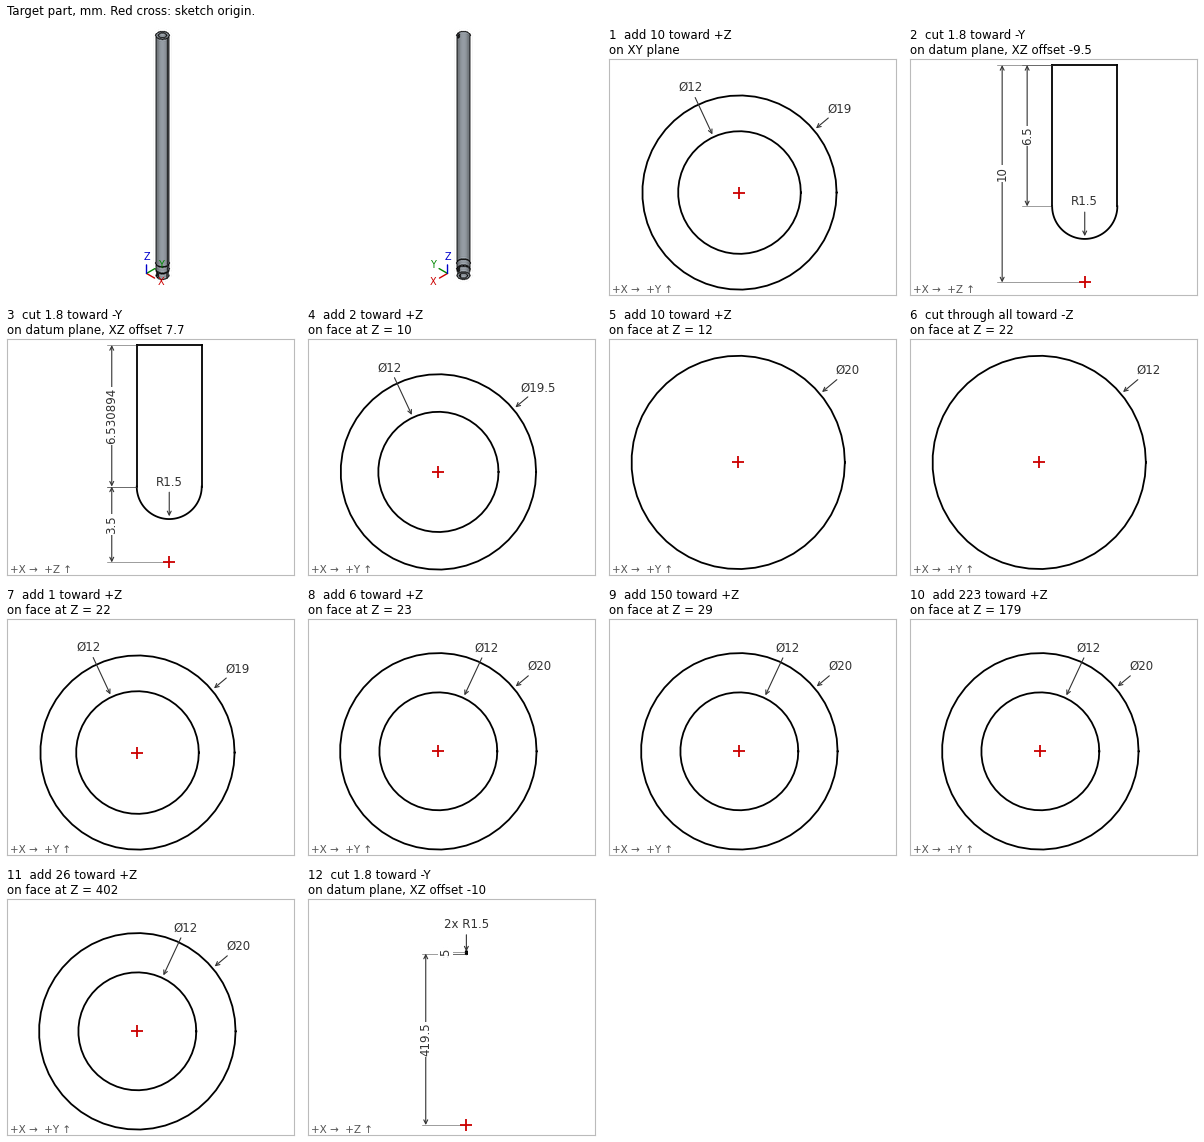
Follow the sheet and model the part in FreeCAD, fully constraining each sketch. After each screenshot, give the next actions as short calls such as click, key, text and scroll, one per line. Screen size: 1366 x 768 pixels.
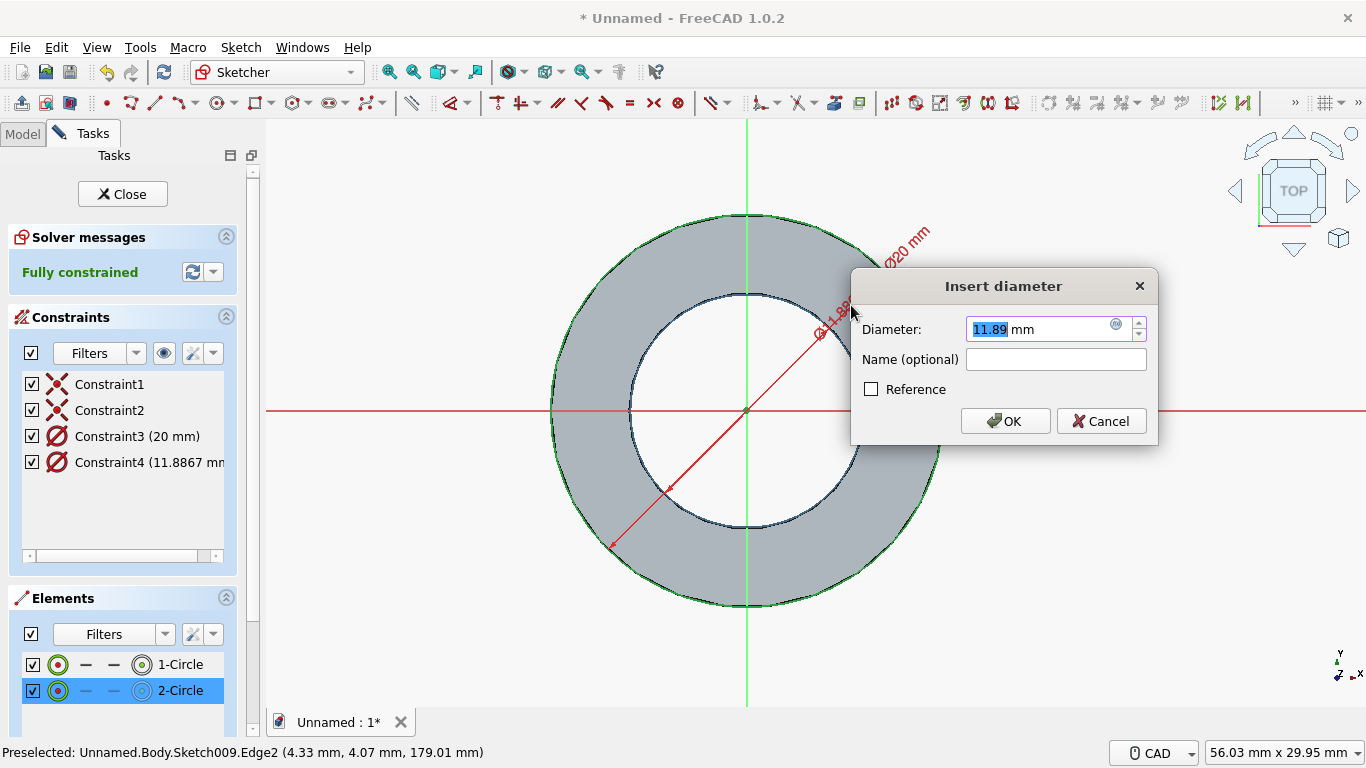
text(12)
key(Return)
key(Escape)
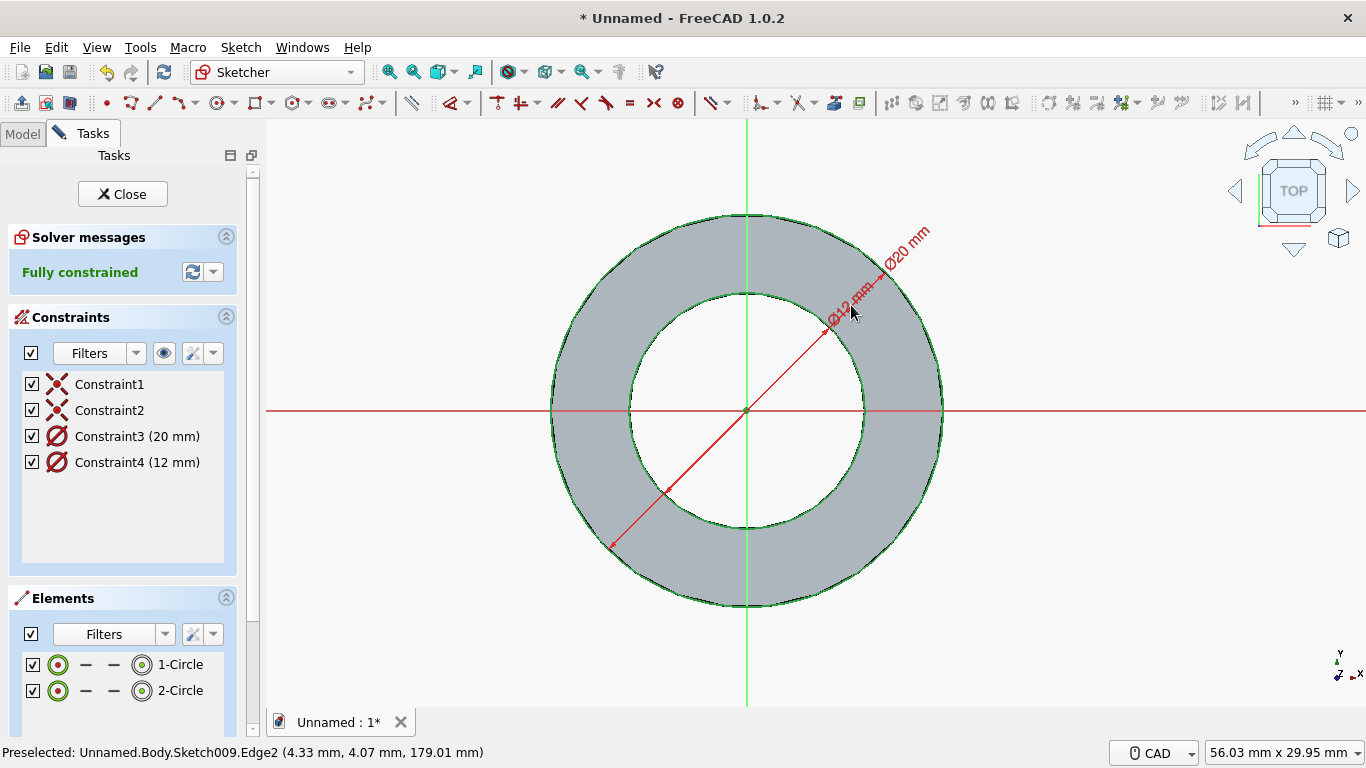
click(123, 194)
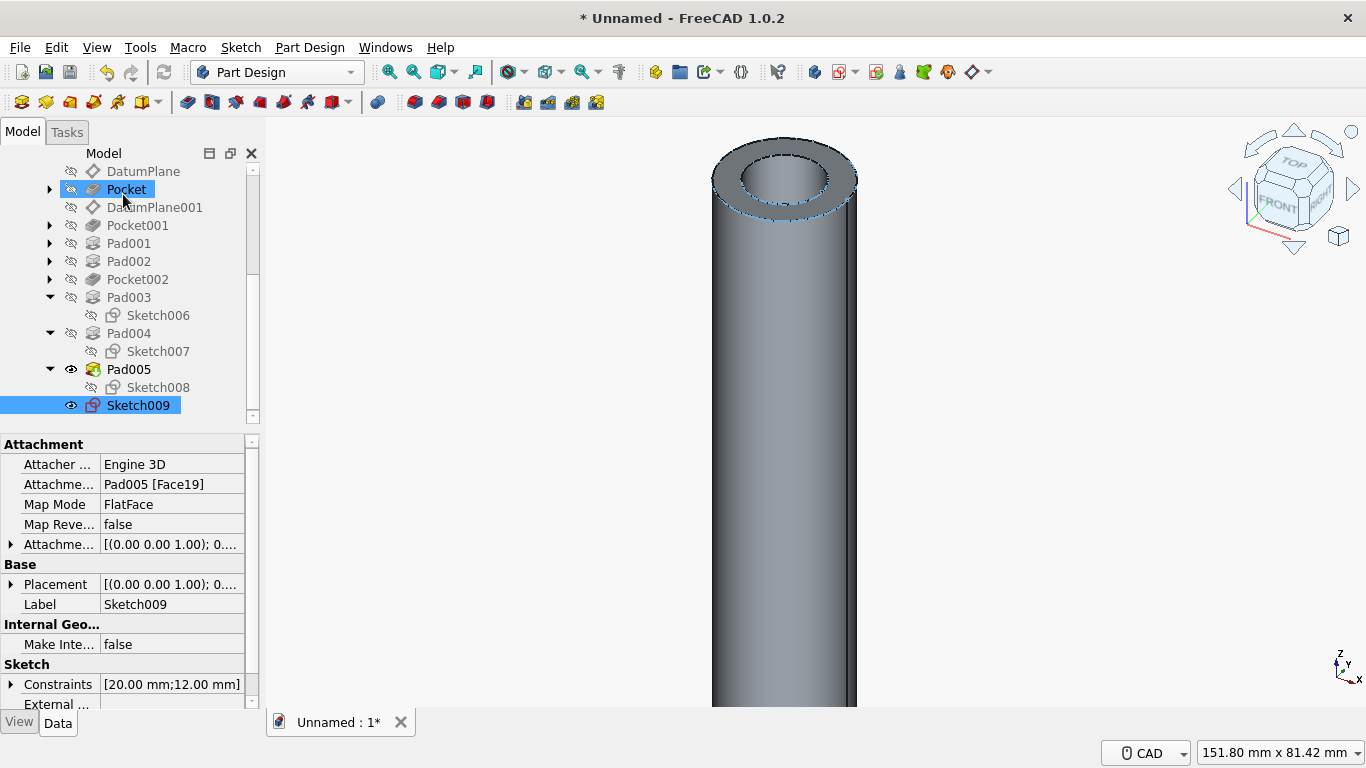
click(22, 102)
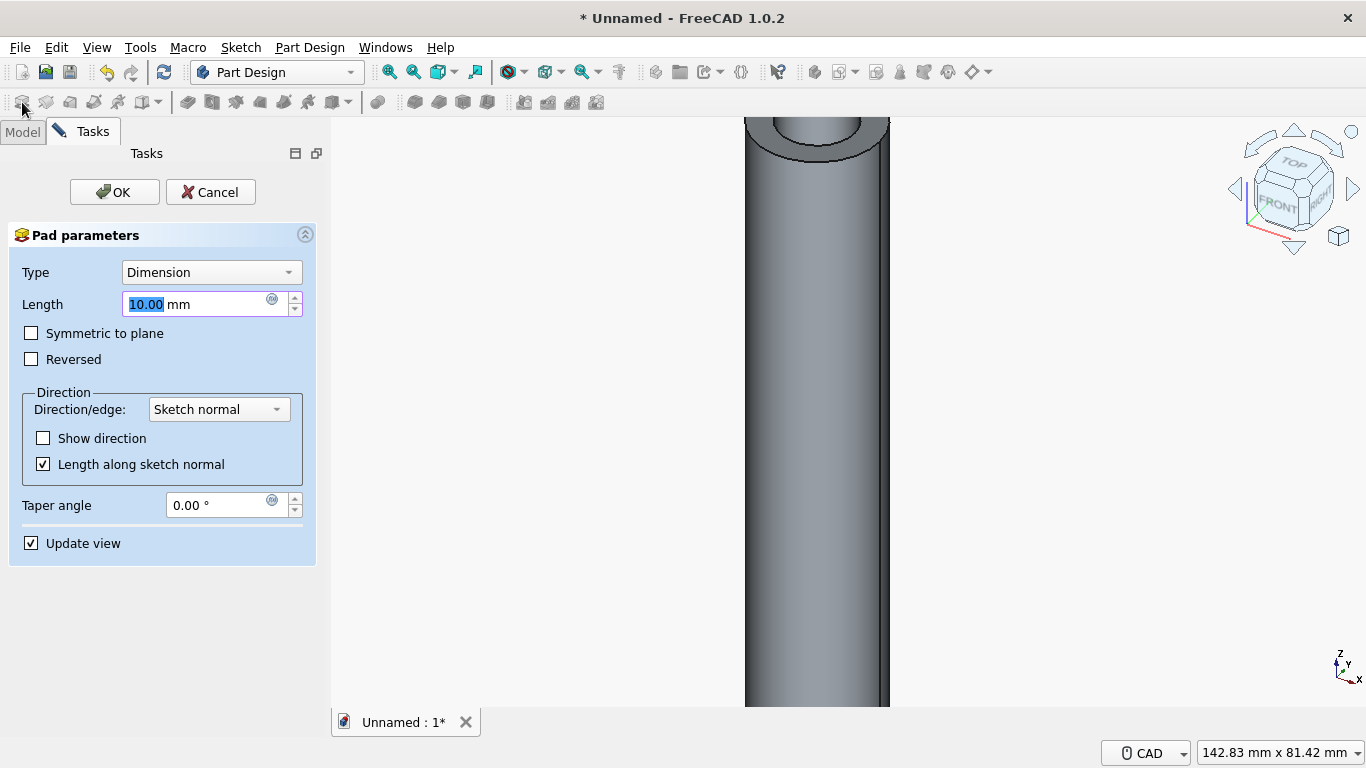
text(223)
key(Tab)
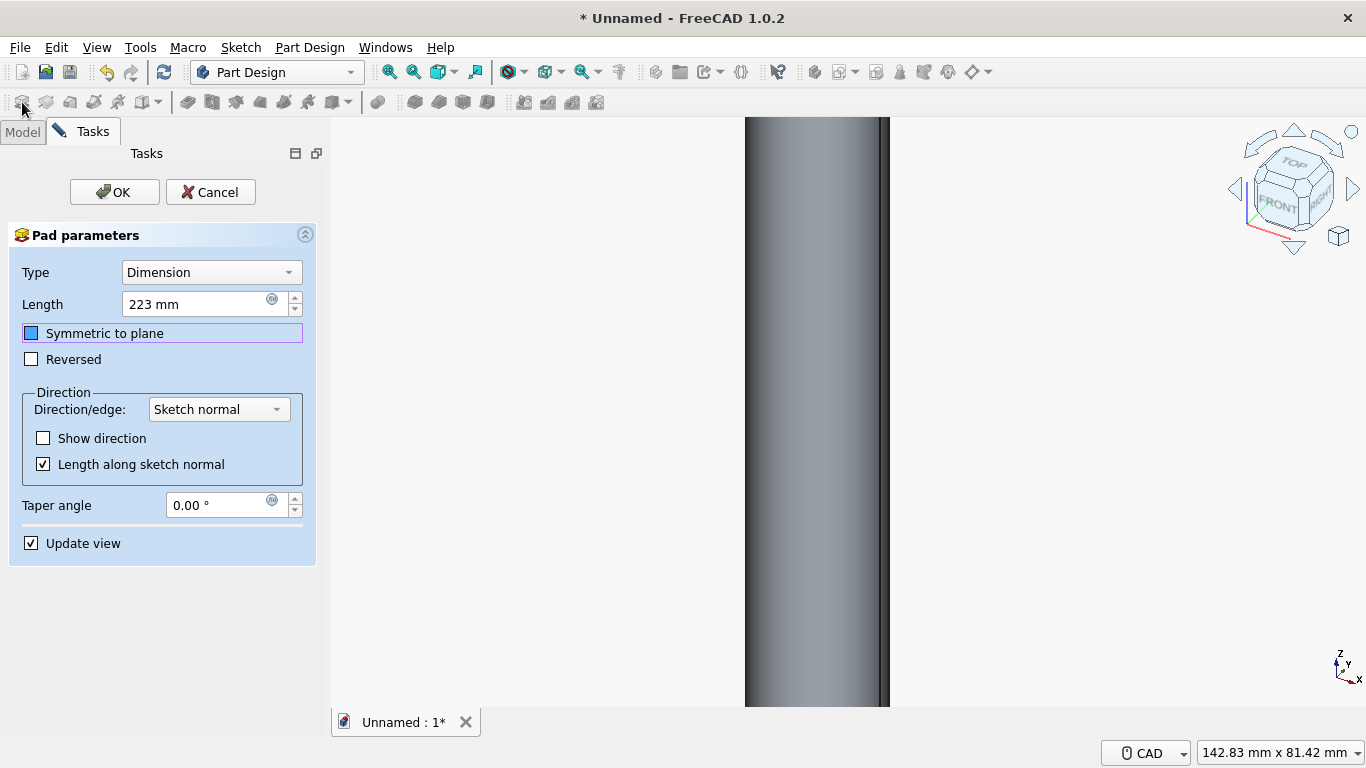
click(115, 192)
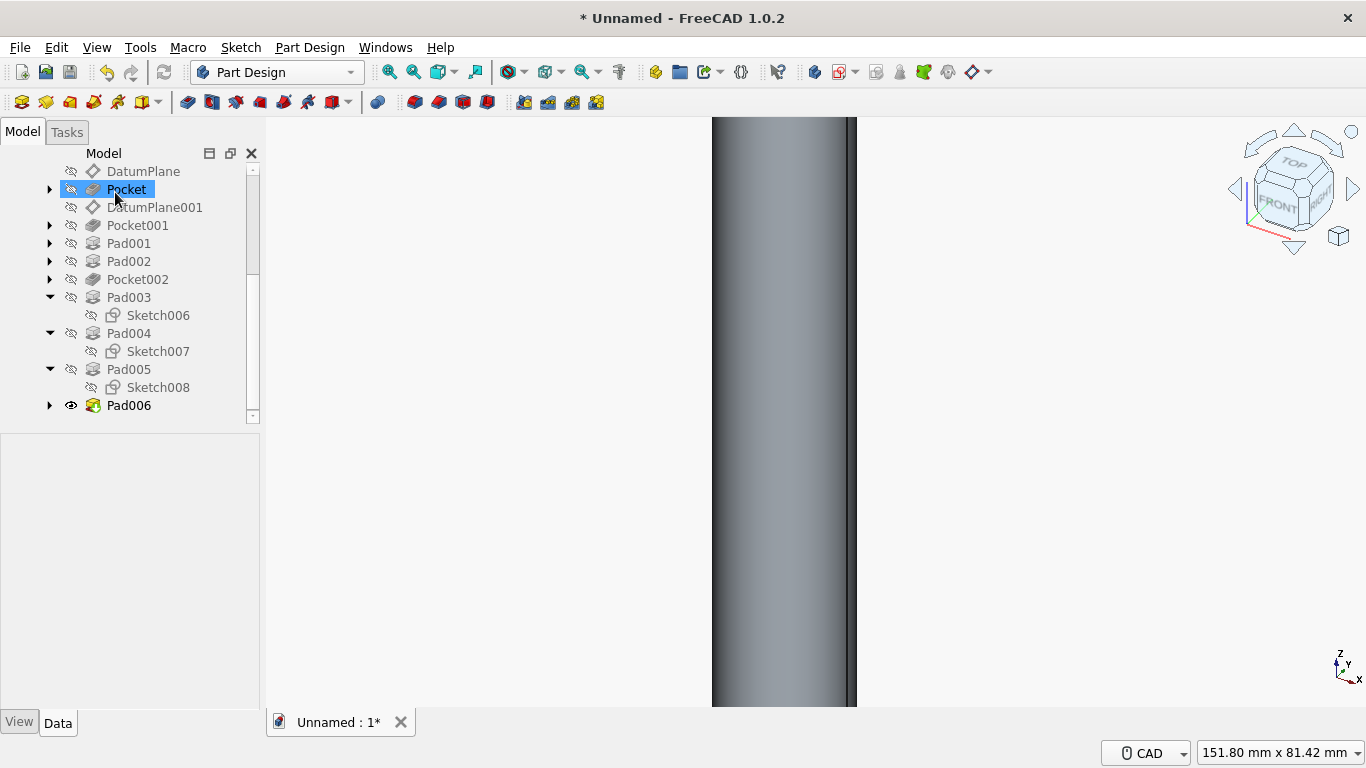
click(390, 72)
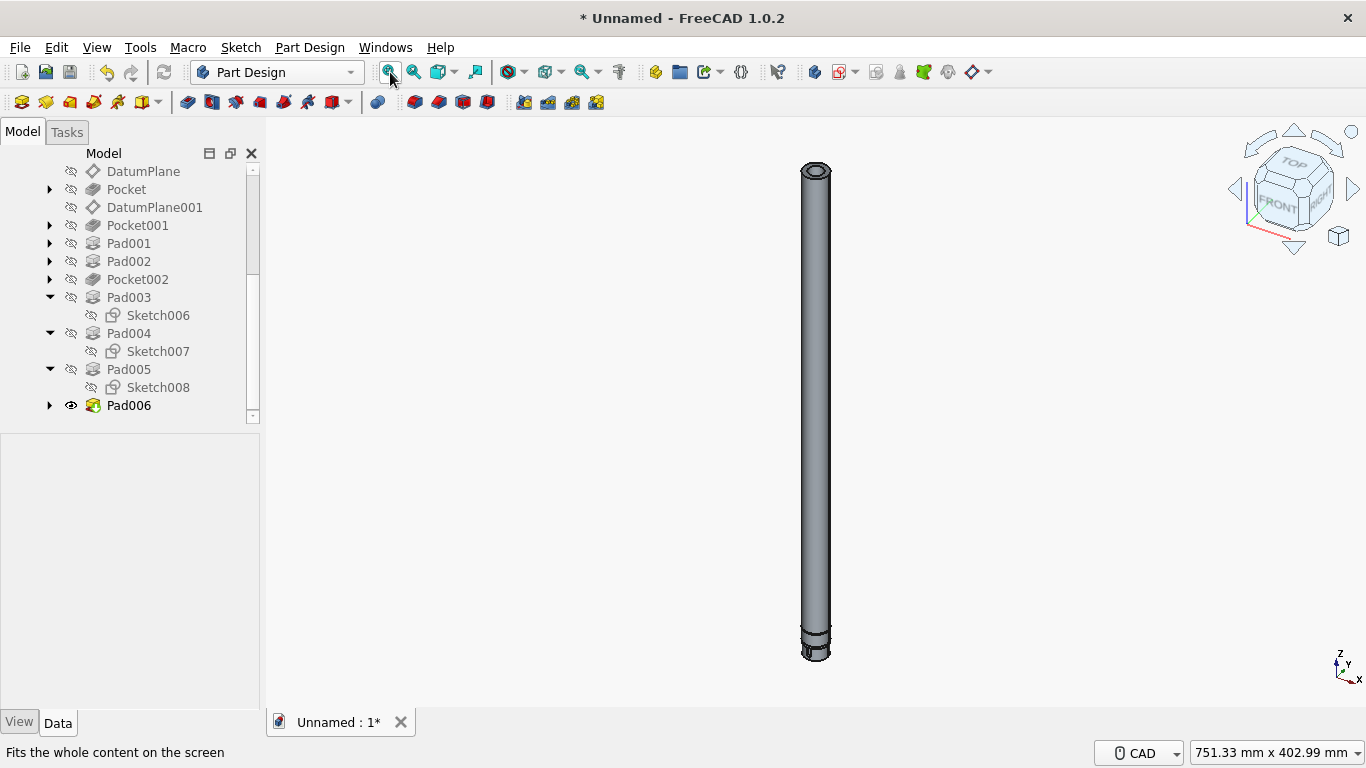
scroll(827, 168, up, 8)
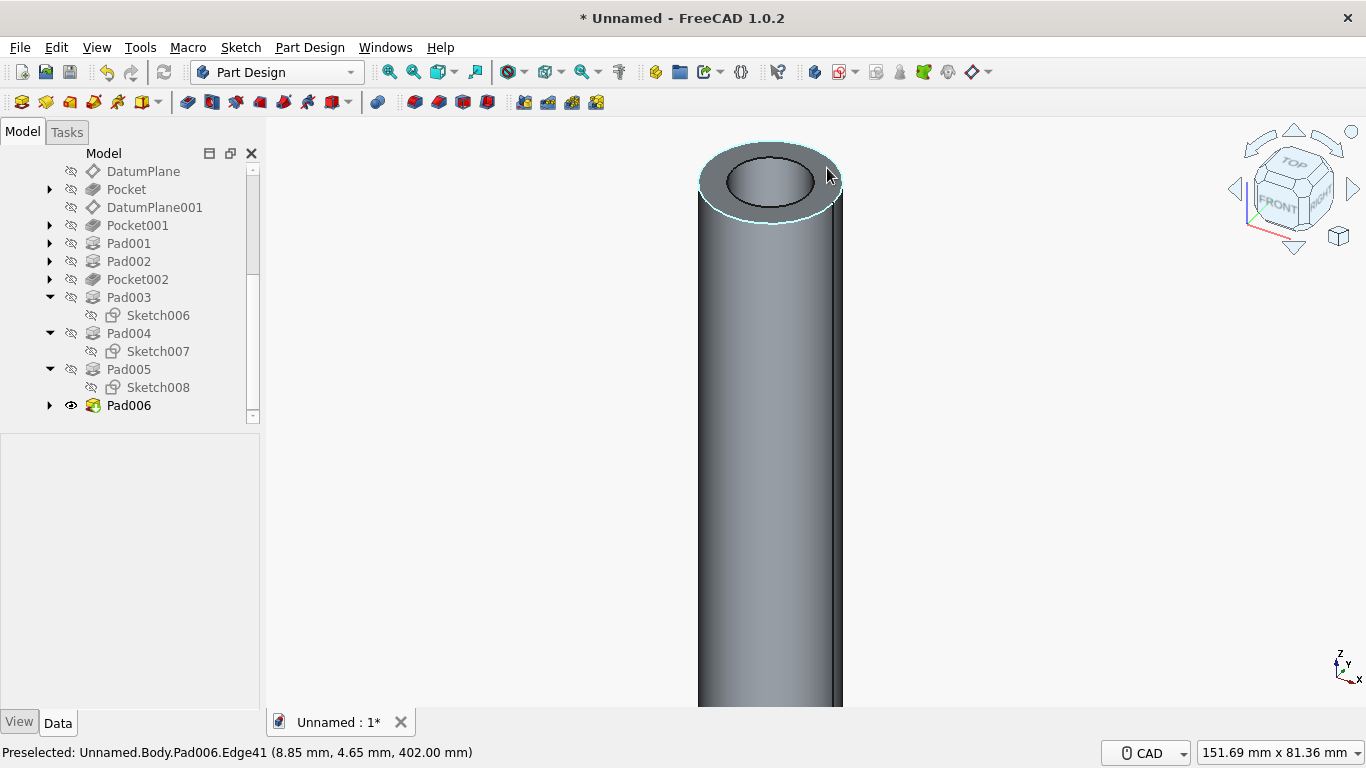
click(827, 173)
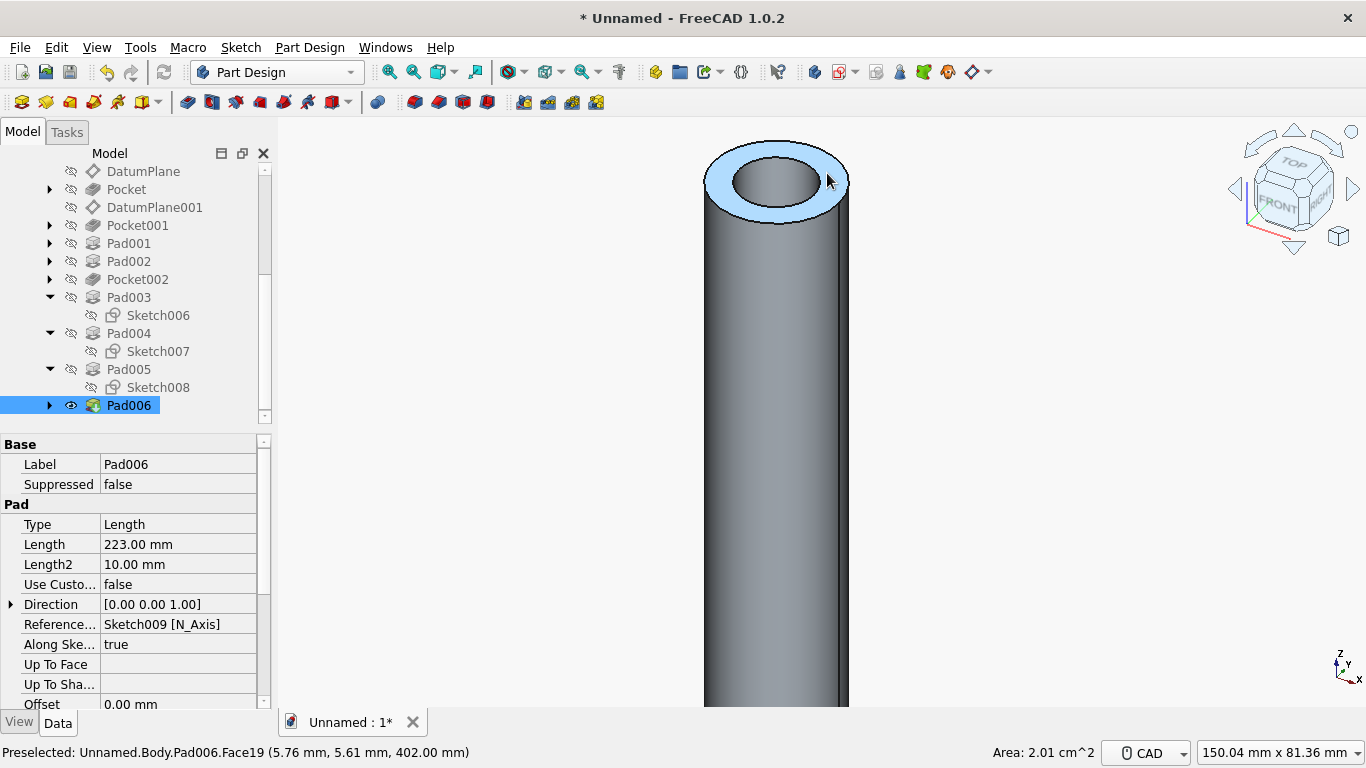
click(840, 72)